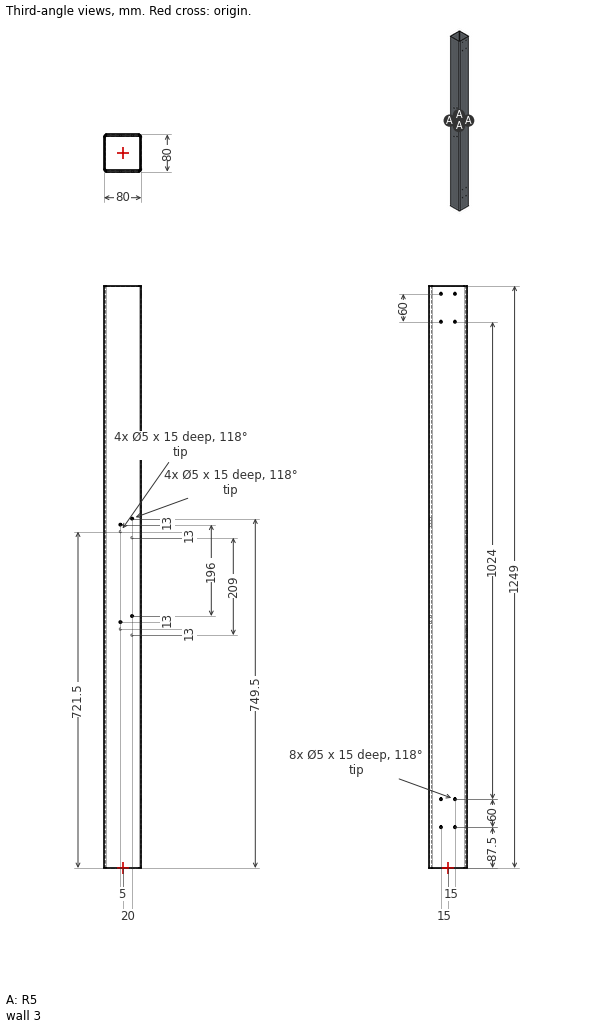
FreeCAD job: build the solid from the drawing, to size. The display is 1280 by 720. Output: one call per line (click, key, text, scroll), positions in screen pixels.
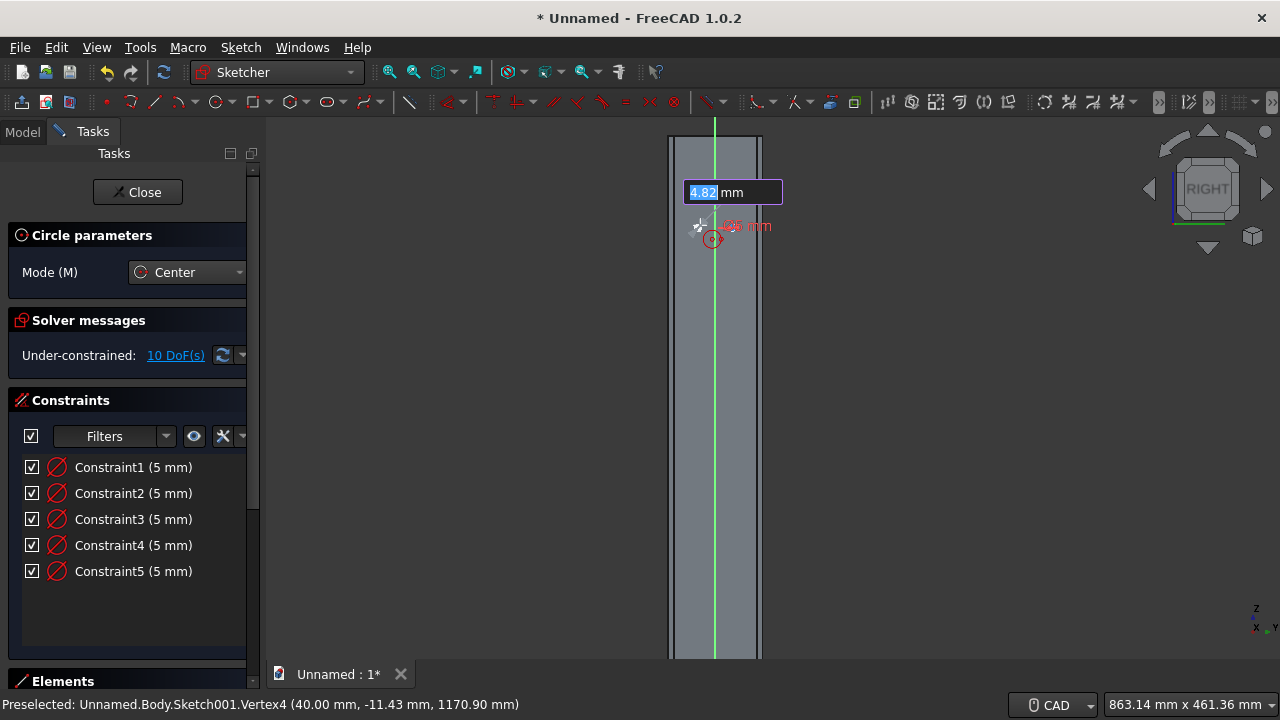
text(5)
key(Return)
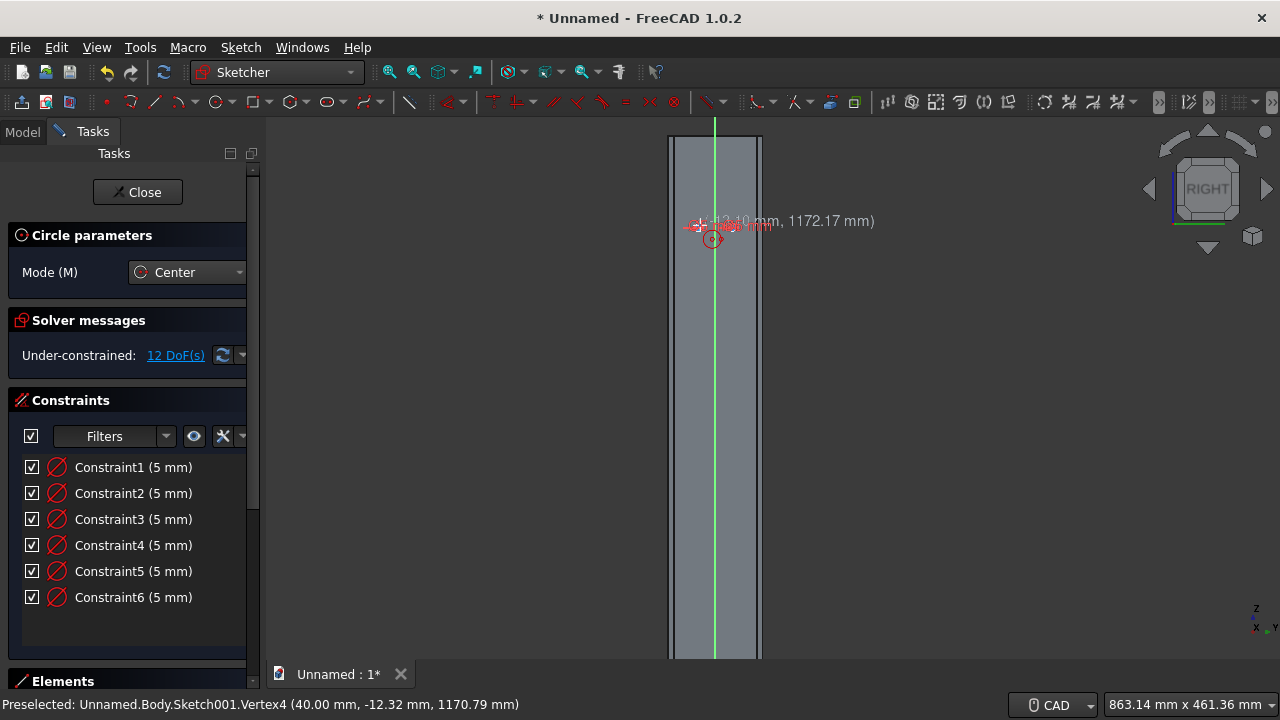
scroll(698, 156, up, 11)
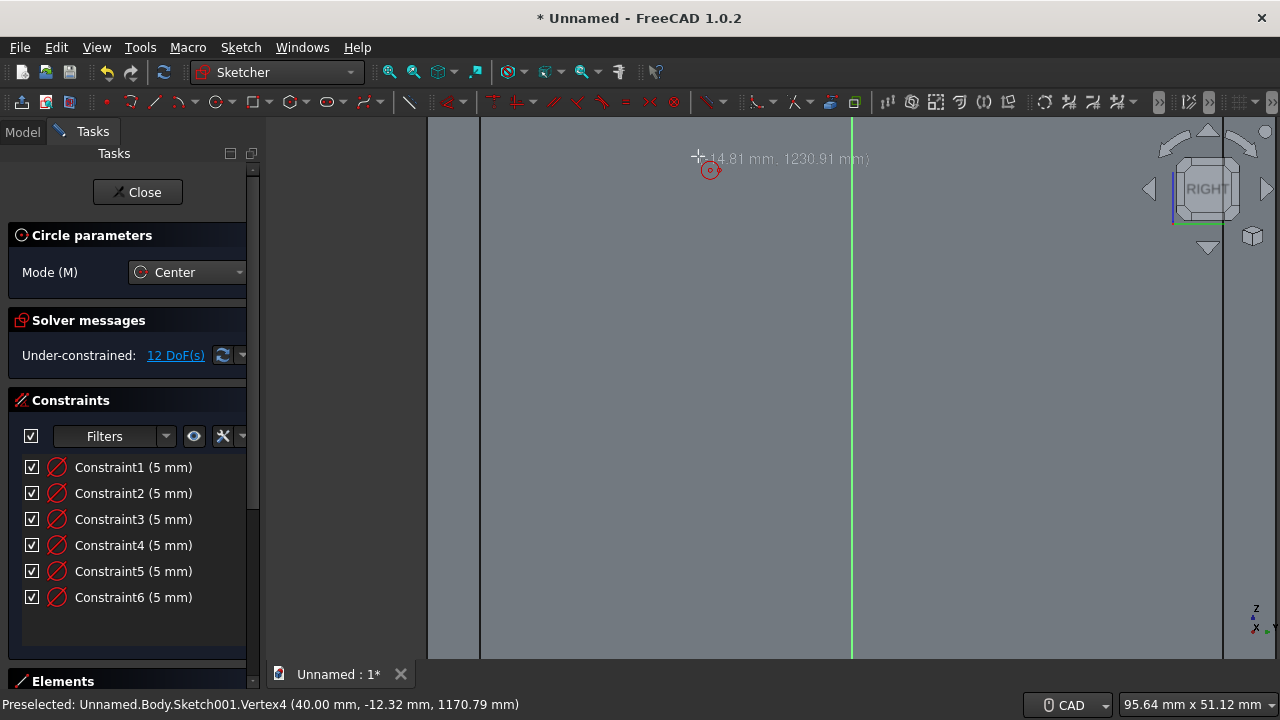
scroll(700, 211, down, 18)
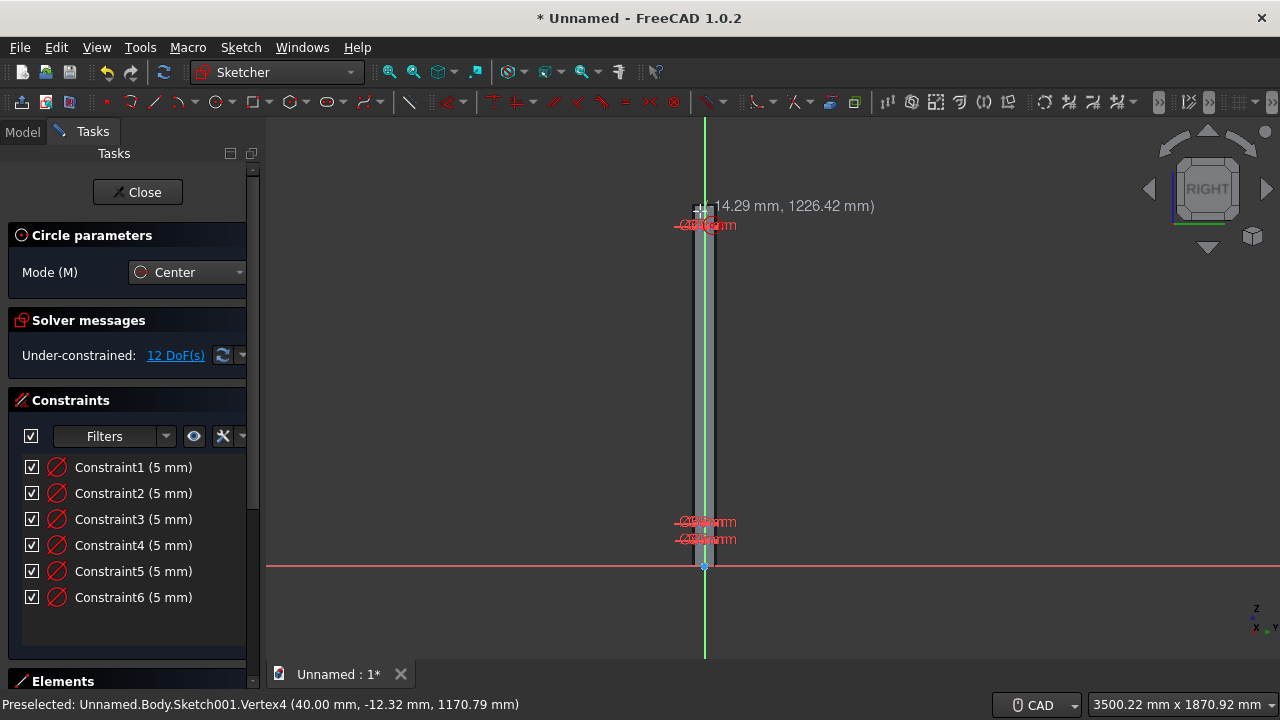
scroll(700, 210, up, 7)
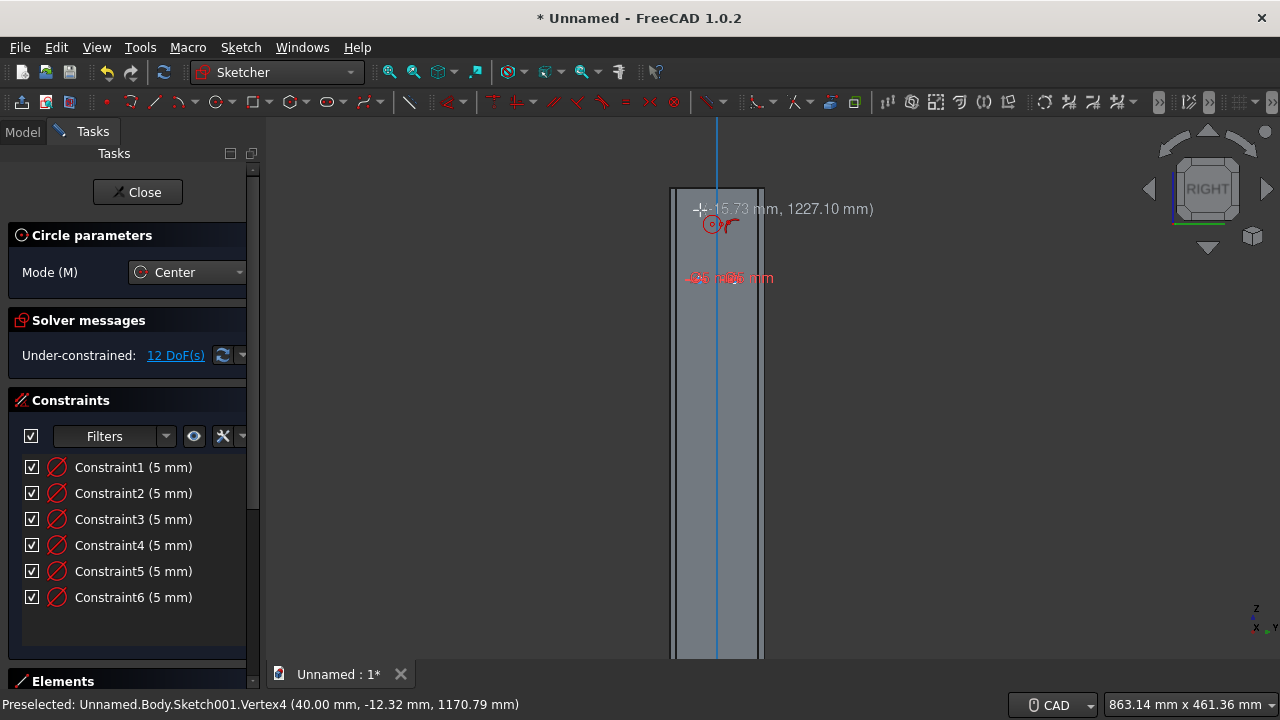
click(700, 208)
move(702, 206)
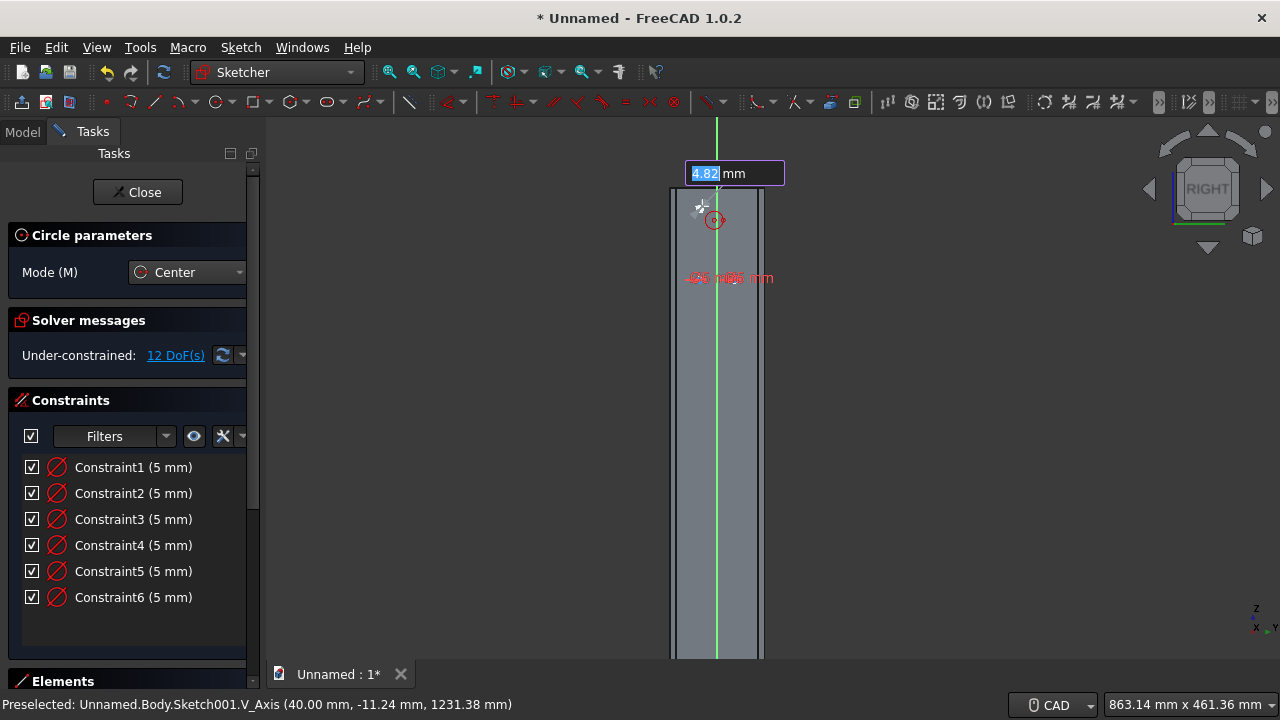
text(5)
key(Return)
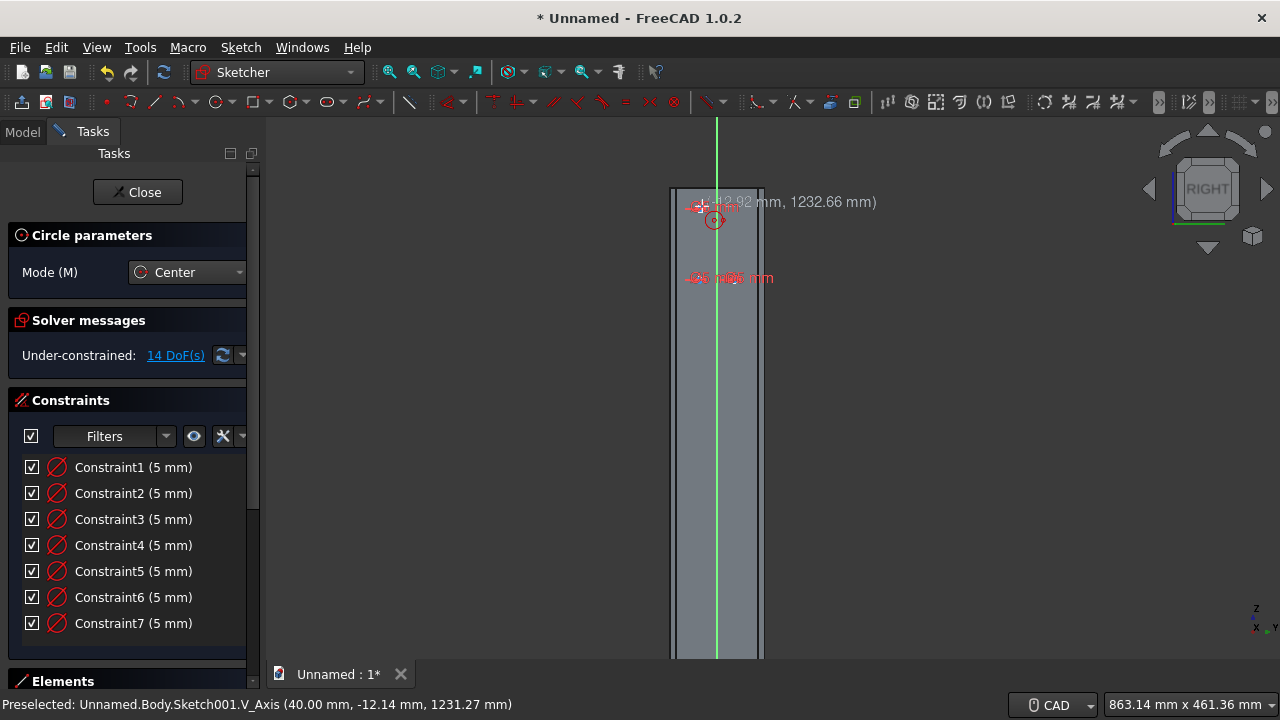
scroll(735, 208, up, 11)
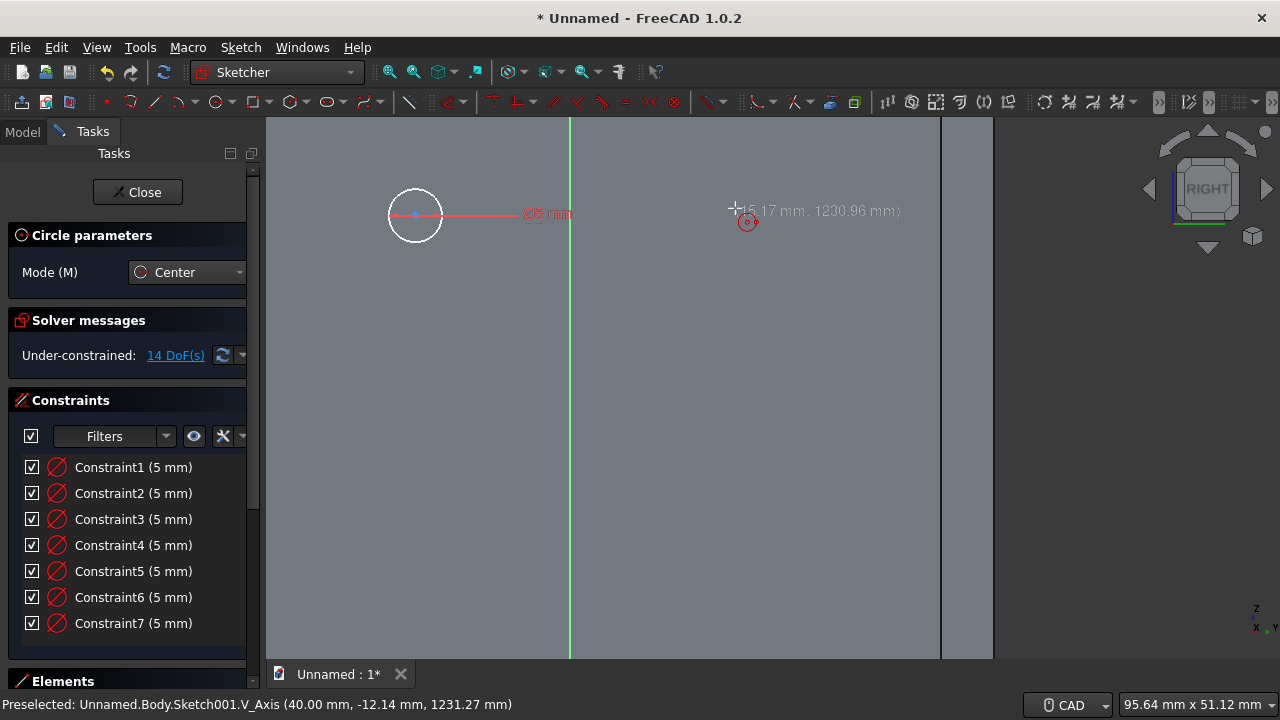
scroll(708, 210, down, 18)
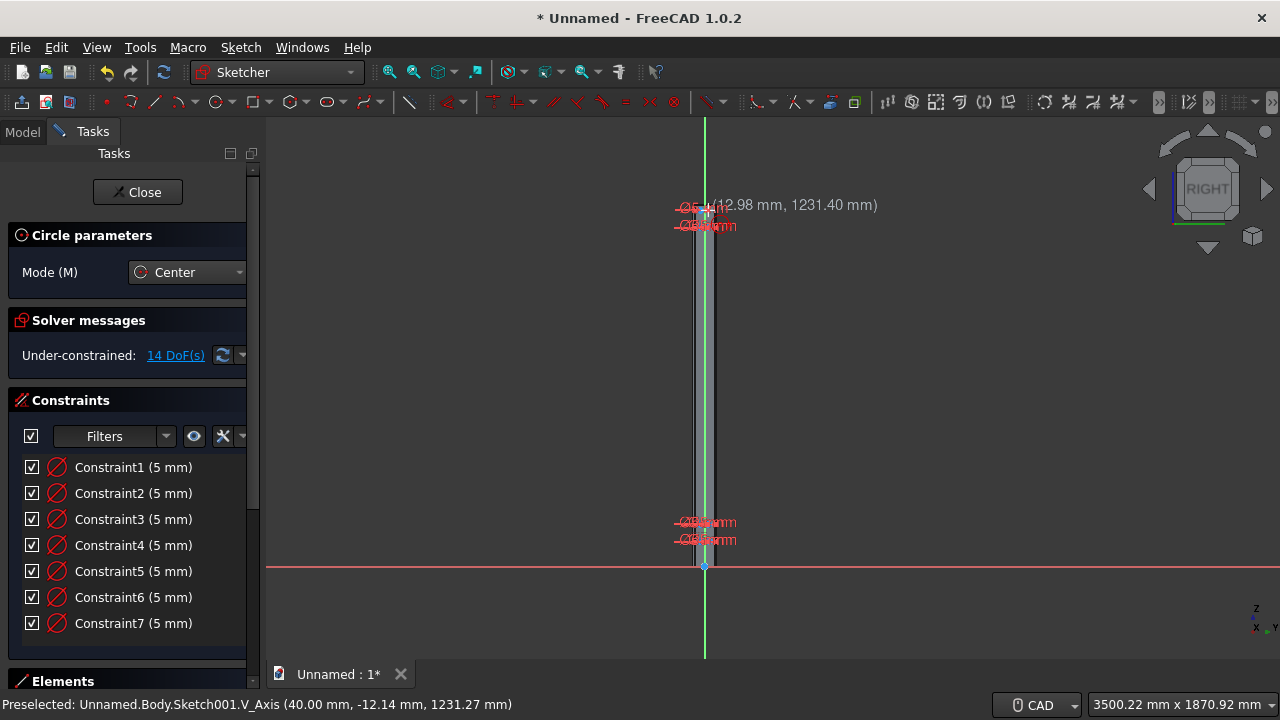
scroll(709, 210, up, 7)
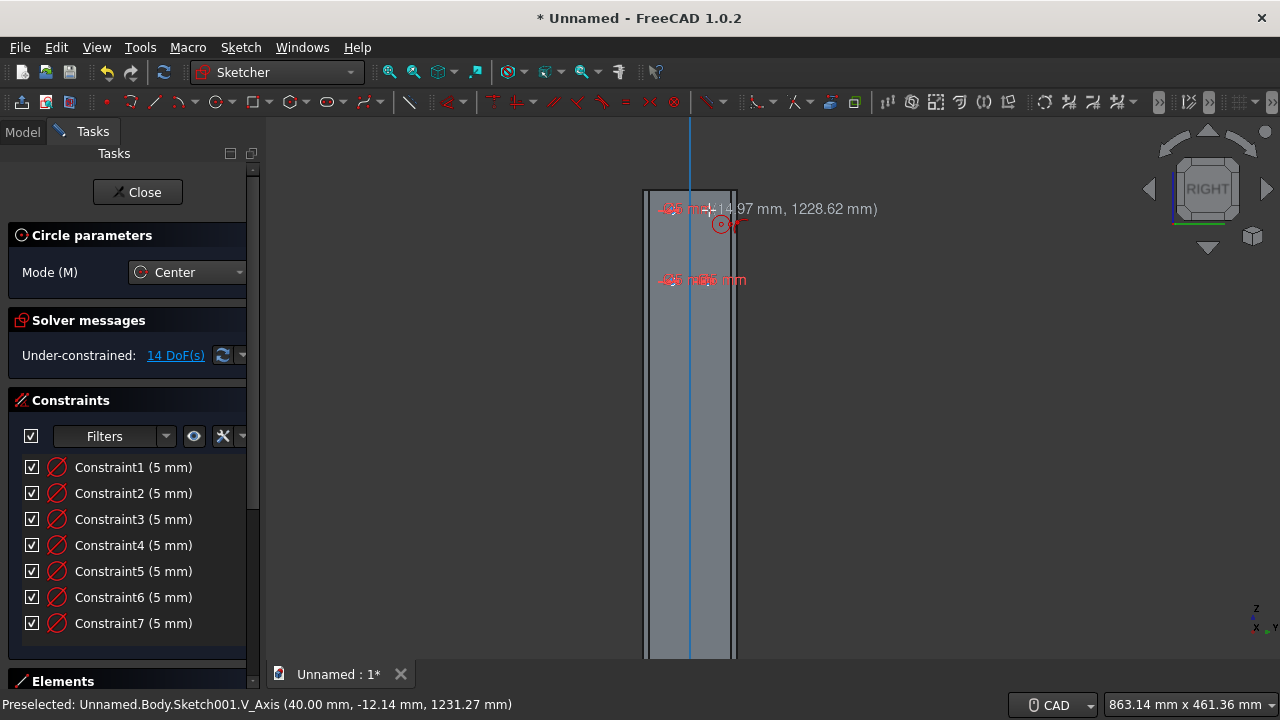
click(708, 210)
move(710, 208)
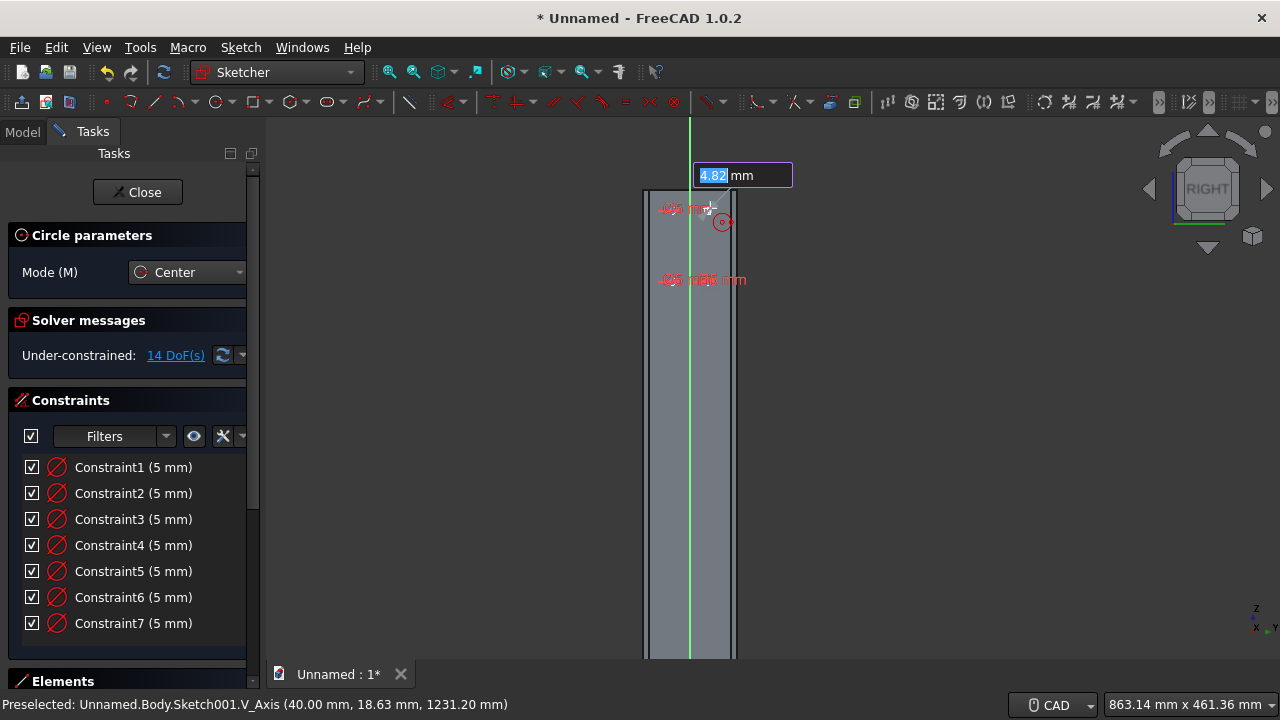
text(5)
key(Return)
key(Escape)